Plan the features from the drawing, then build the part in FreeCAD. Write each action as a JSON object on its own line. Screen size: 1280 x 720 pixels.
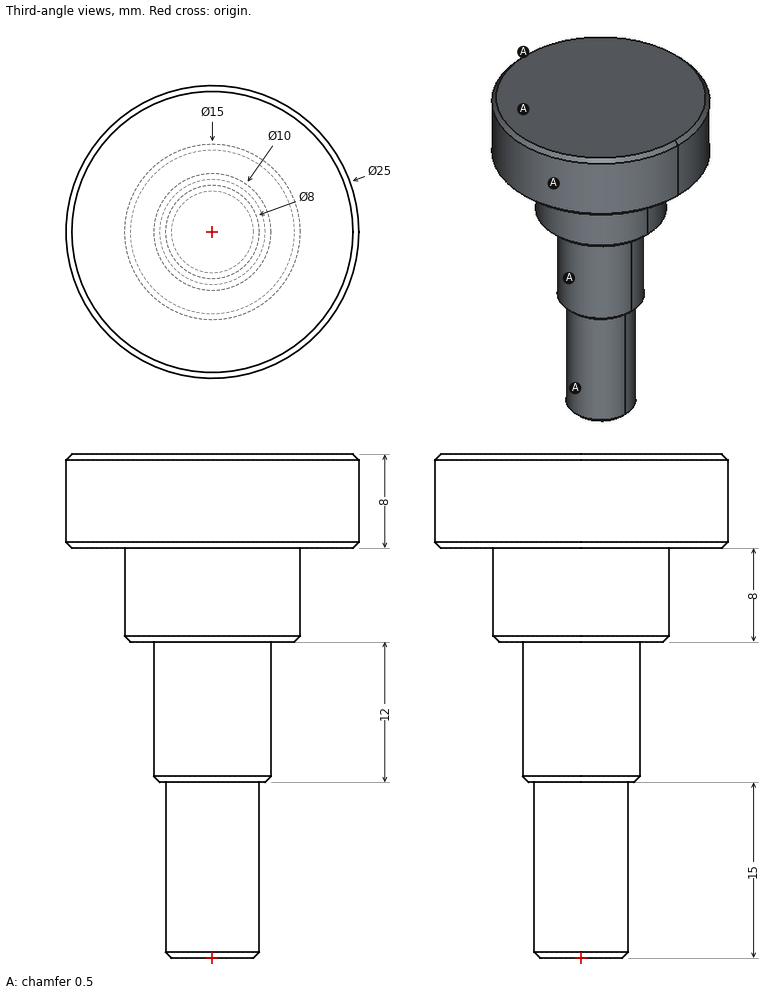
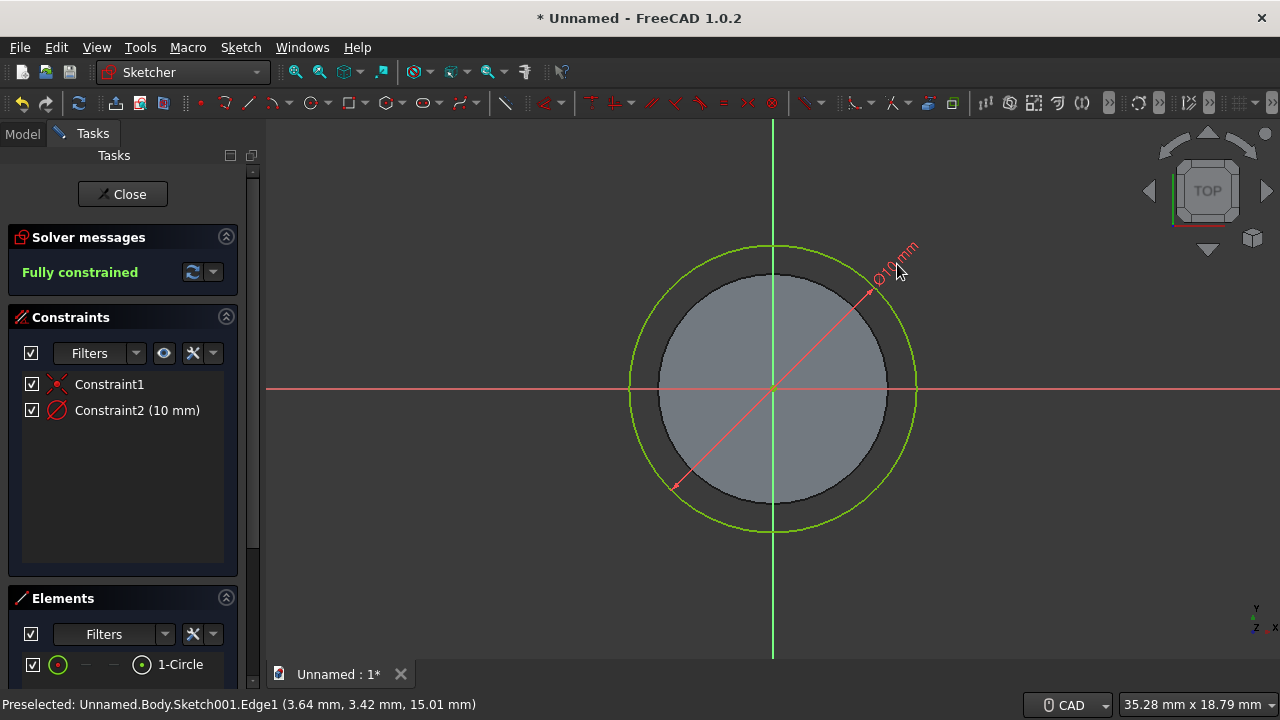
{"action": "left_click", "coordinate": [123, 194]}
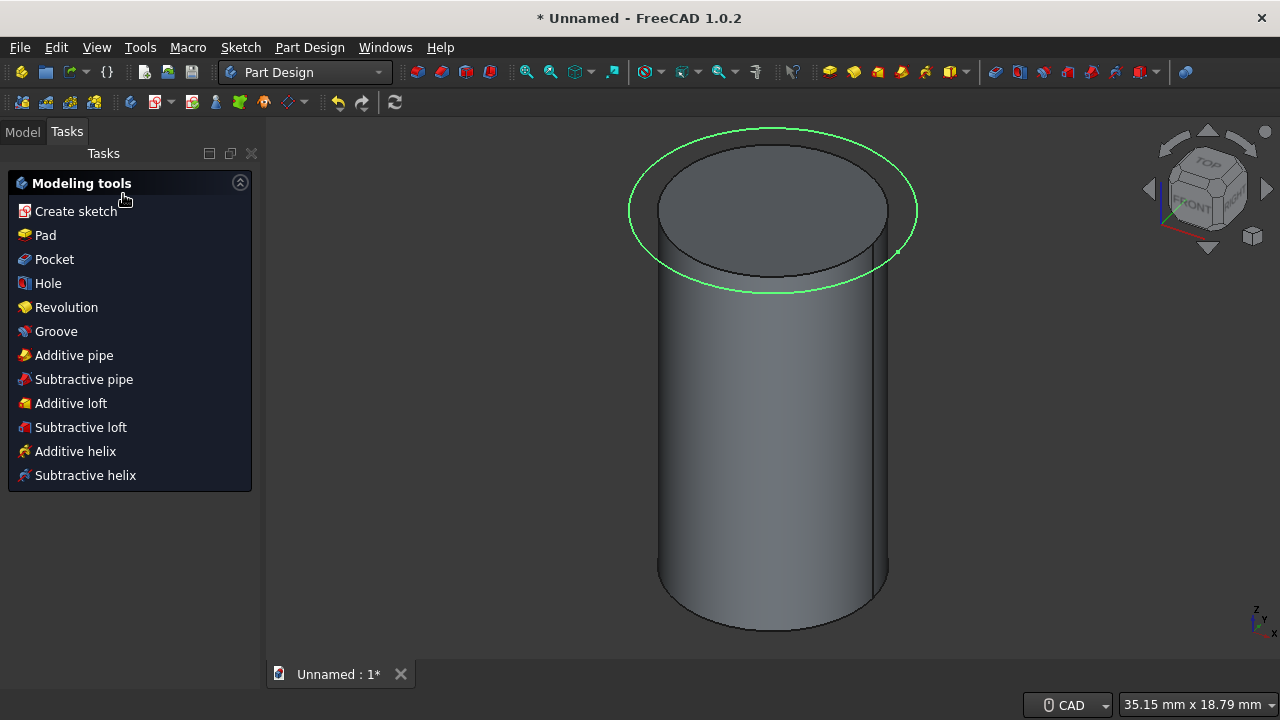
{"action": "left_click", "coordinate": [830, 72]}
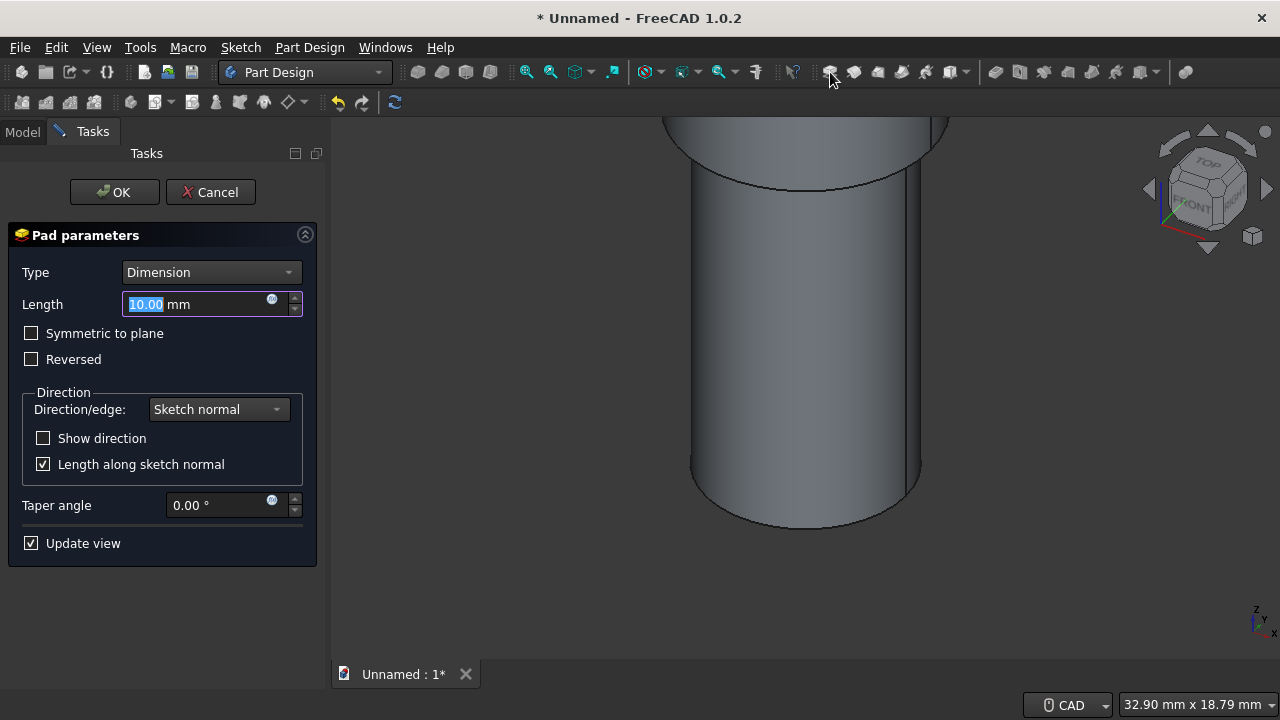
{"action": "type", "text": "12"}
{"action": "key", "text": "Tab"}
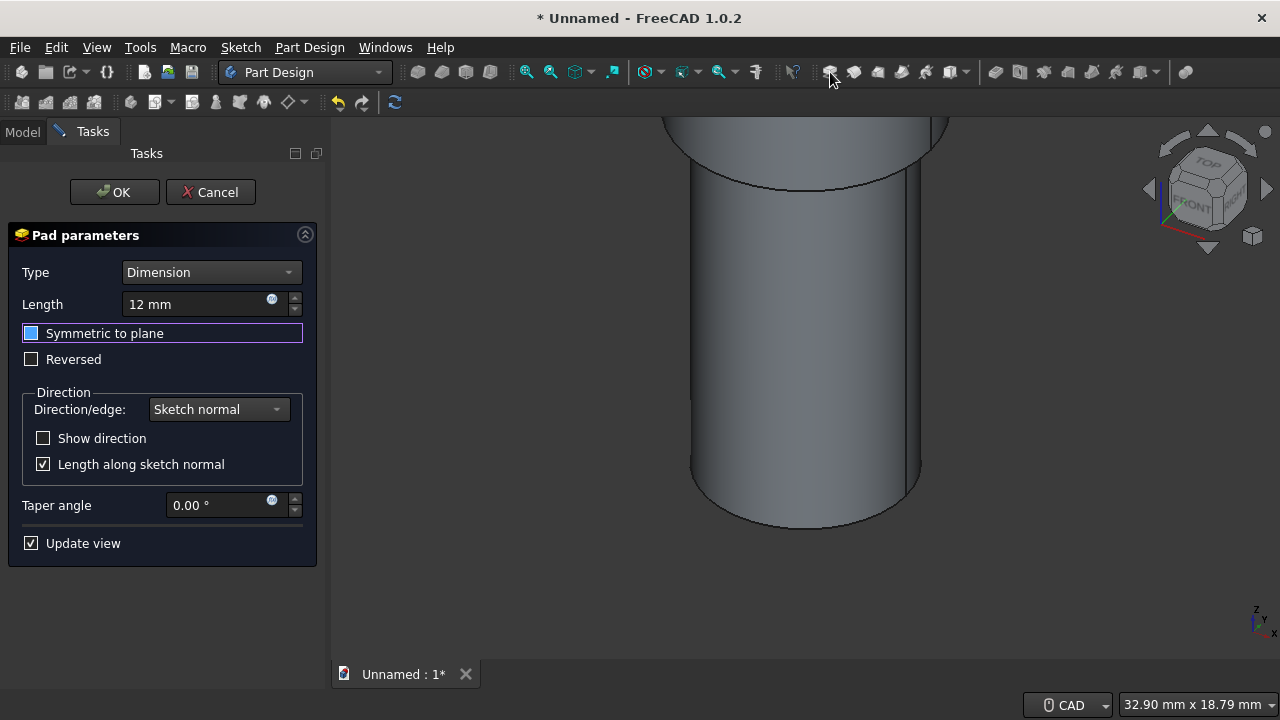
{"action": "left_click", "coordinate": [115, 192]}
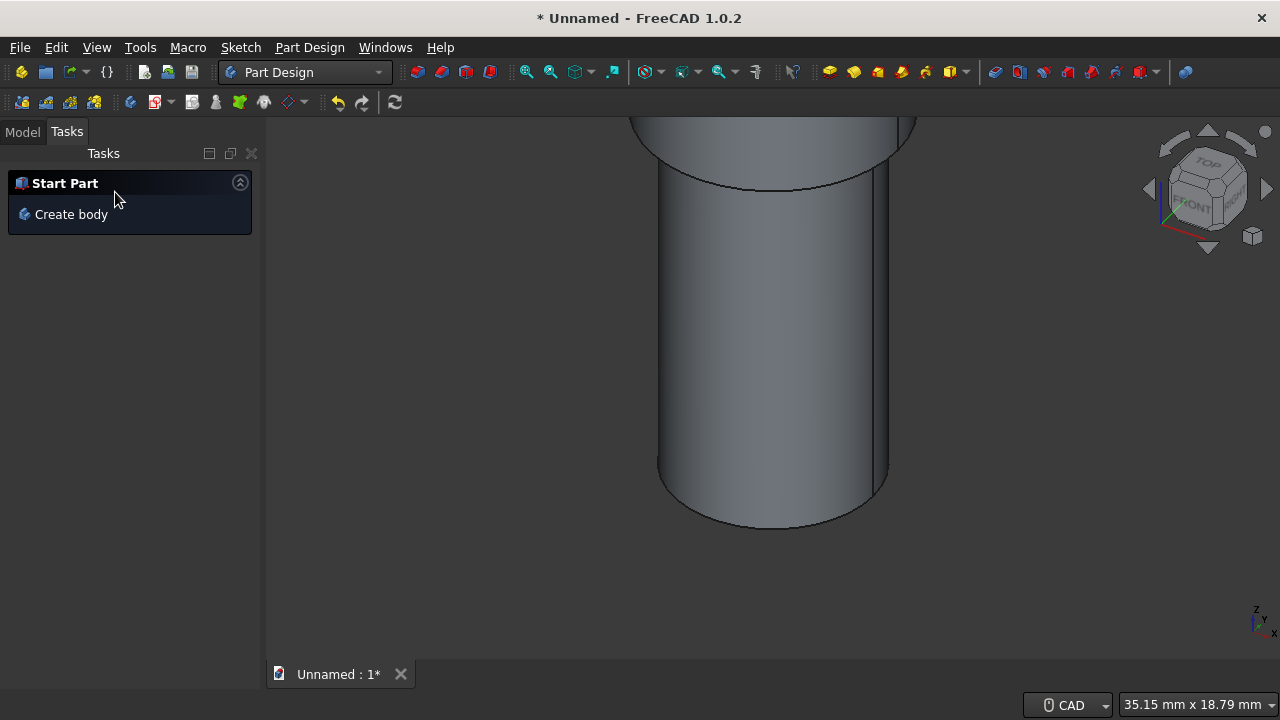
{"action": "left_click", "coordinate": [528, 72]}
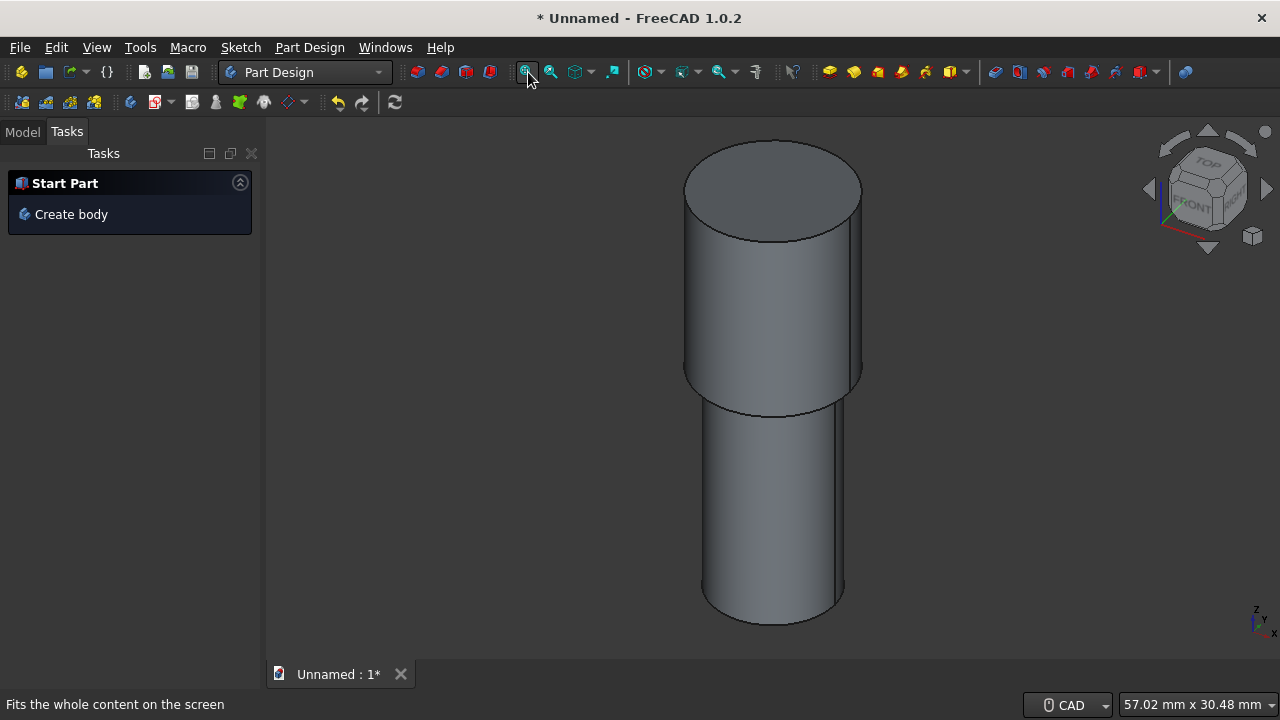
{"action": "left_click", "coordinate": [773, 190]}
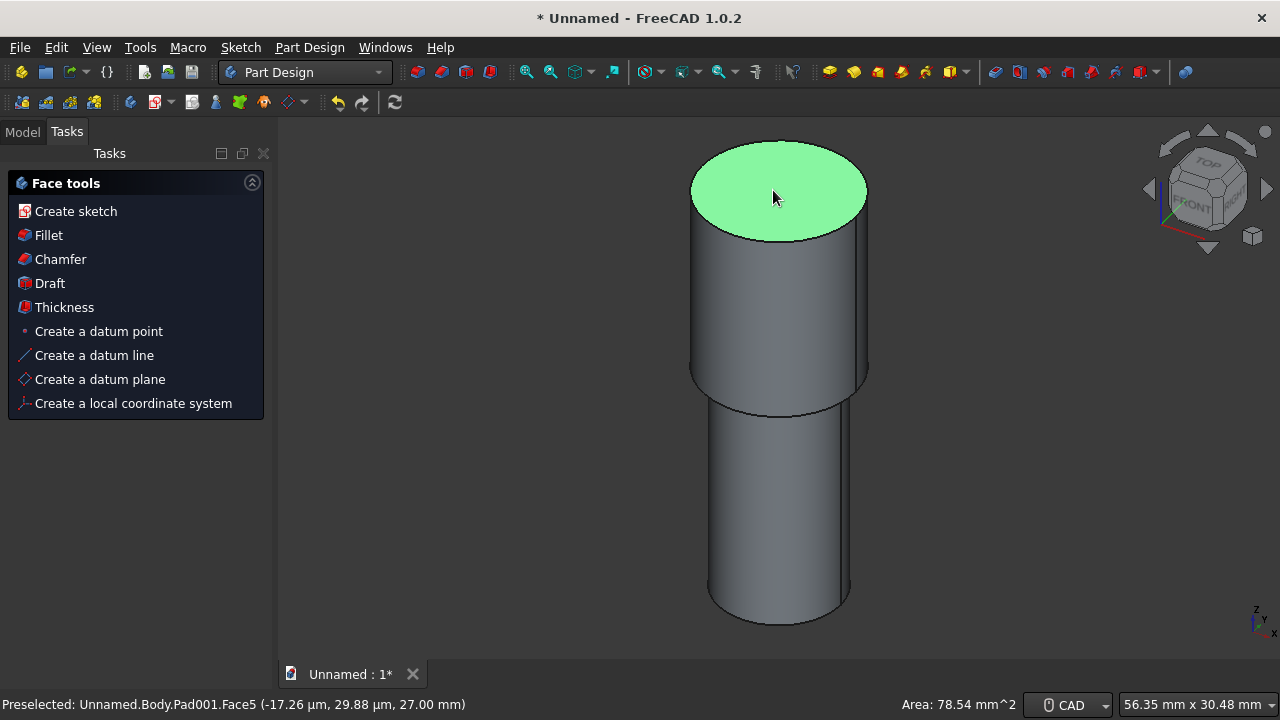
{"action": "left_click", "coordinate": [156, 102]}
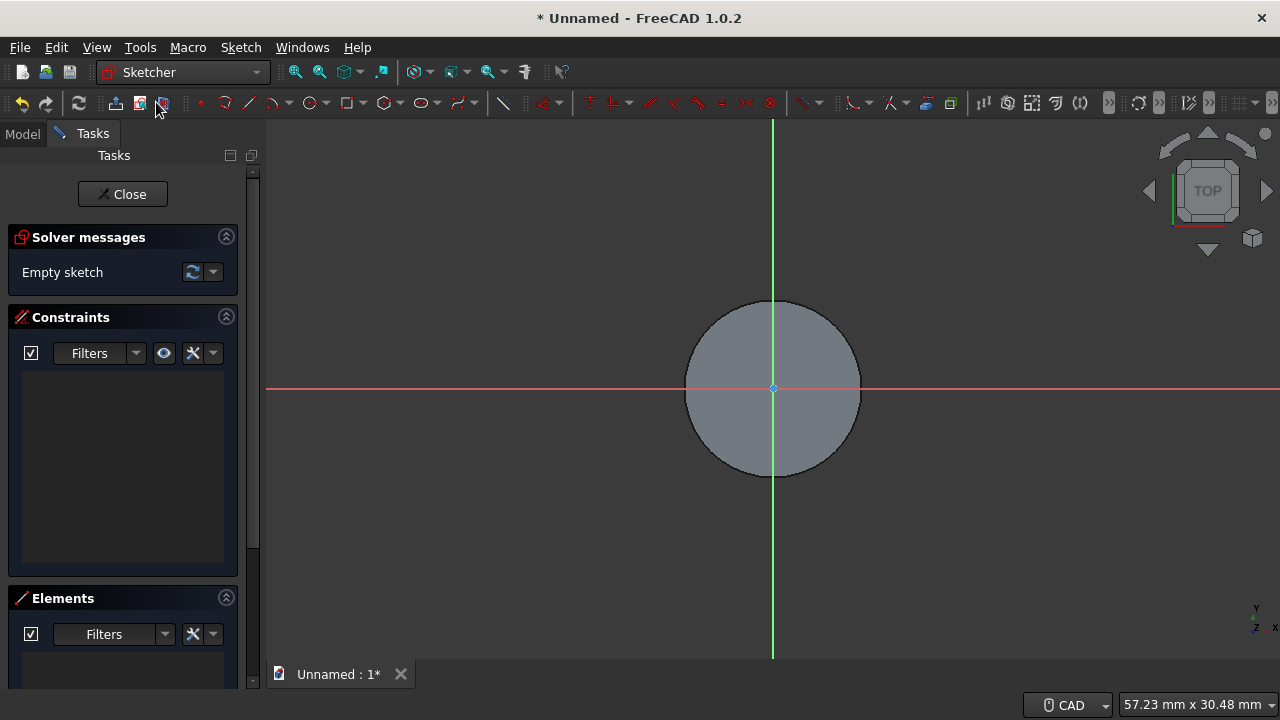
{"action": "left_click", "coordinate": [310, 104]}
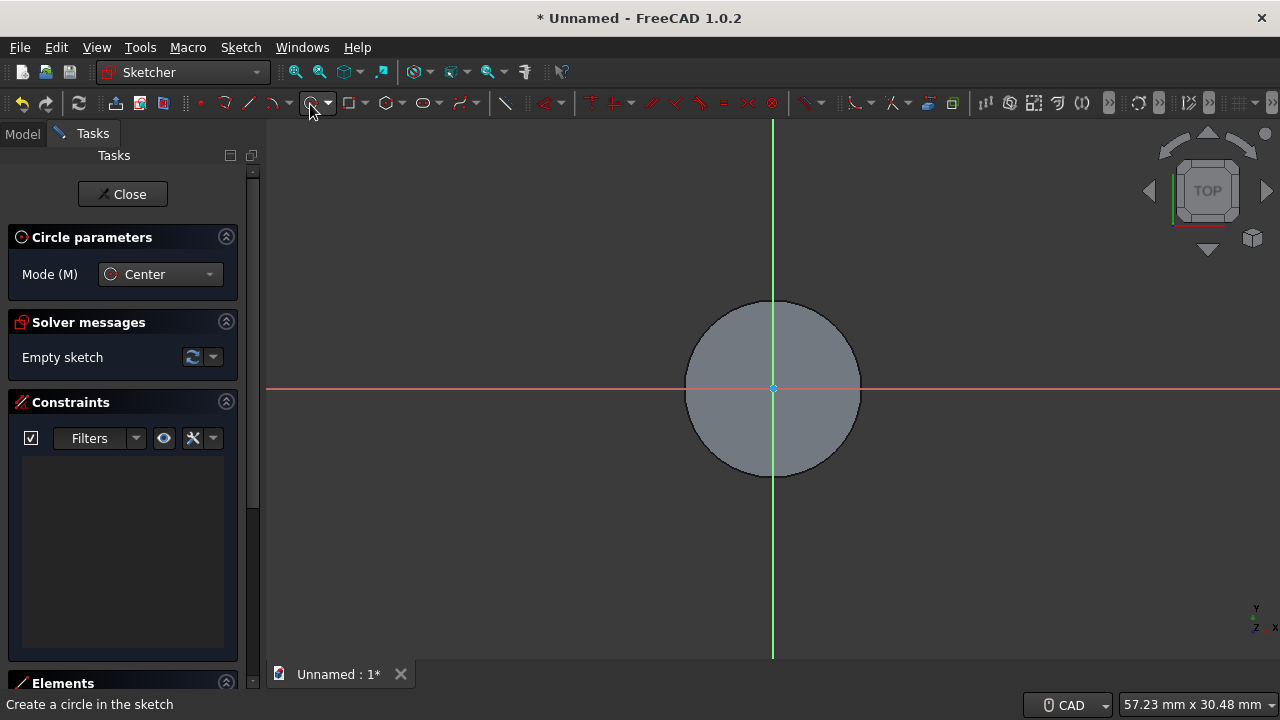
{"action": "left_click", "coordinate": [773, 389]}
{"action": "left_click", "coordinate": [867, 295]}
{"action": "key", "text": "Escape"}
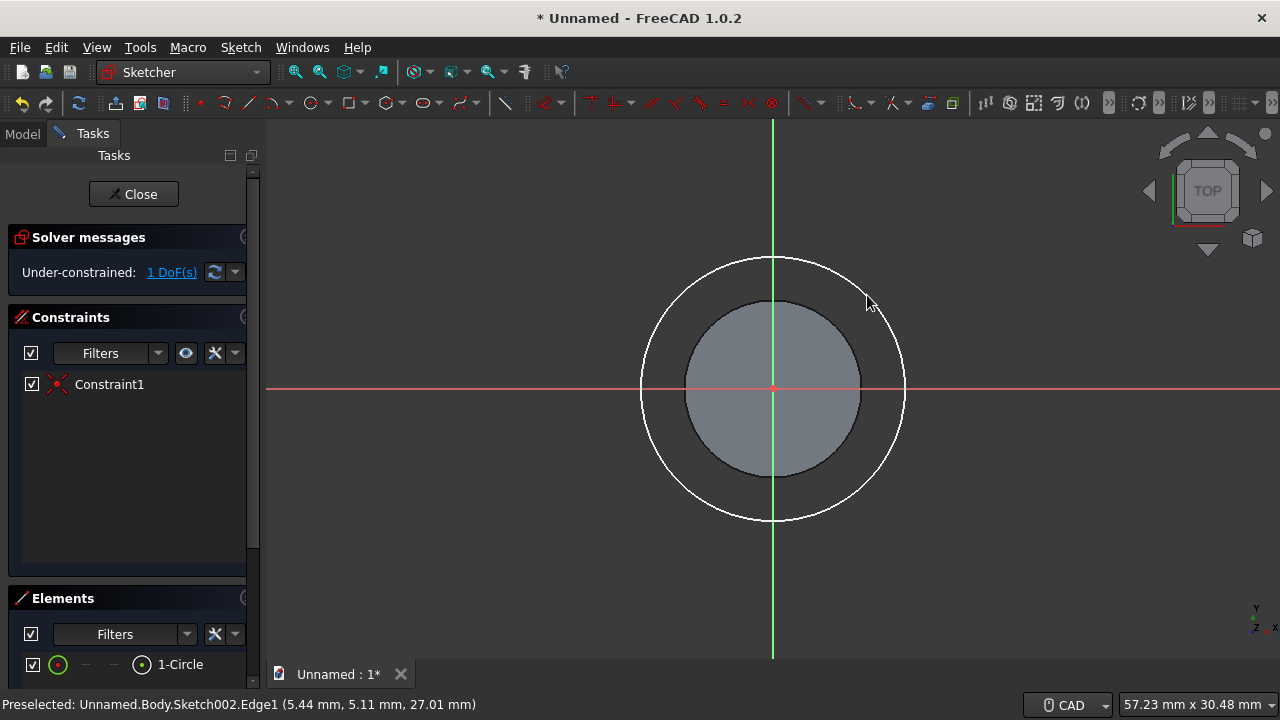
{"action": "left_click", "coordinate": [544, 104]}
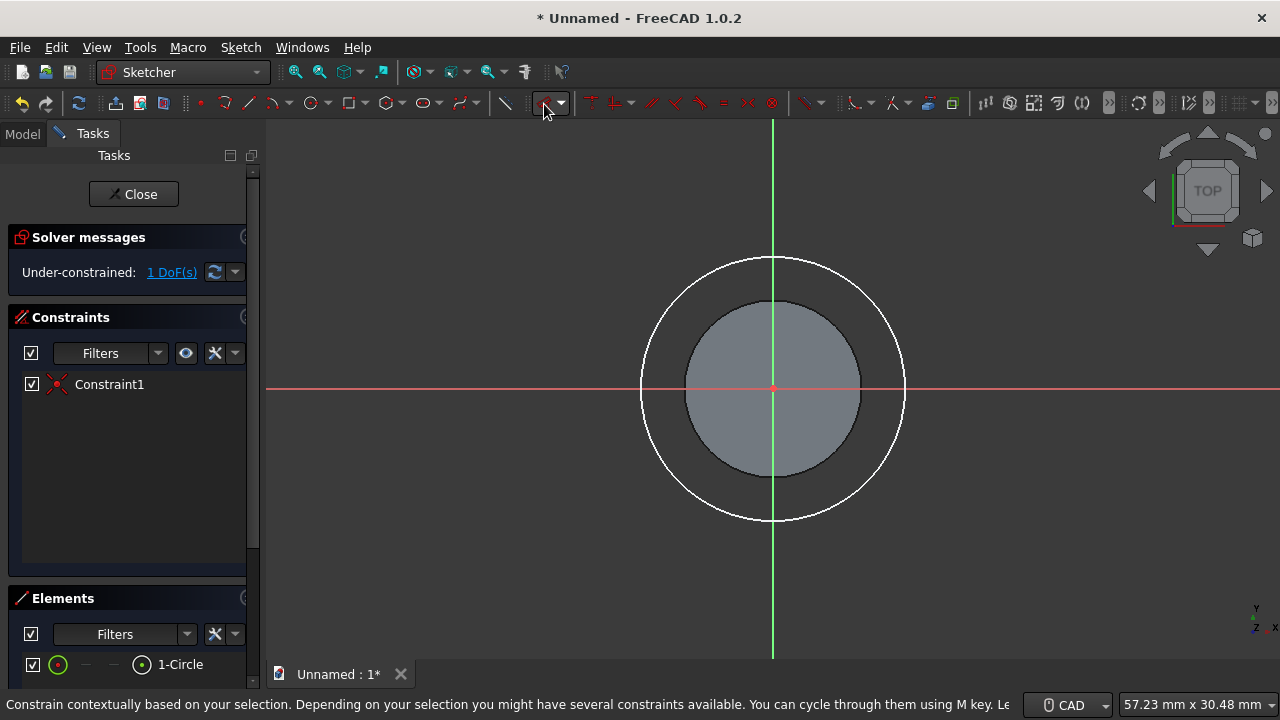
{"action": "left_click", "coordinate": [866, 295]}
{"action": "left_click", "coordinate": [889, 272]}